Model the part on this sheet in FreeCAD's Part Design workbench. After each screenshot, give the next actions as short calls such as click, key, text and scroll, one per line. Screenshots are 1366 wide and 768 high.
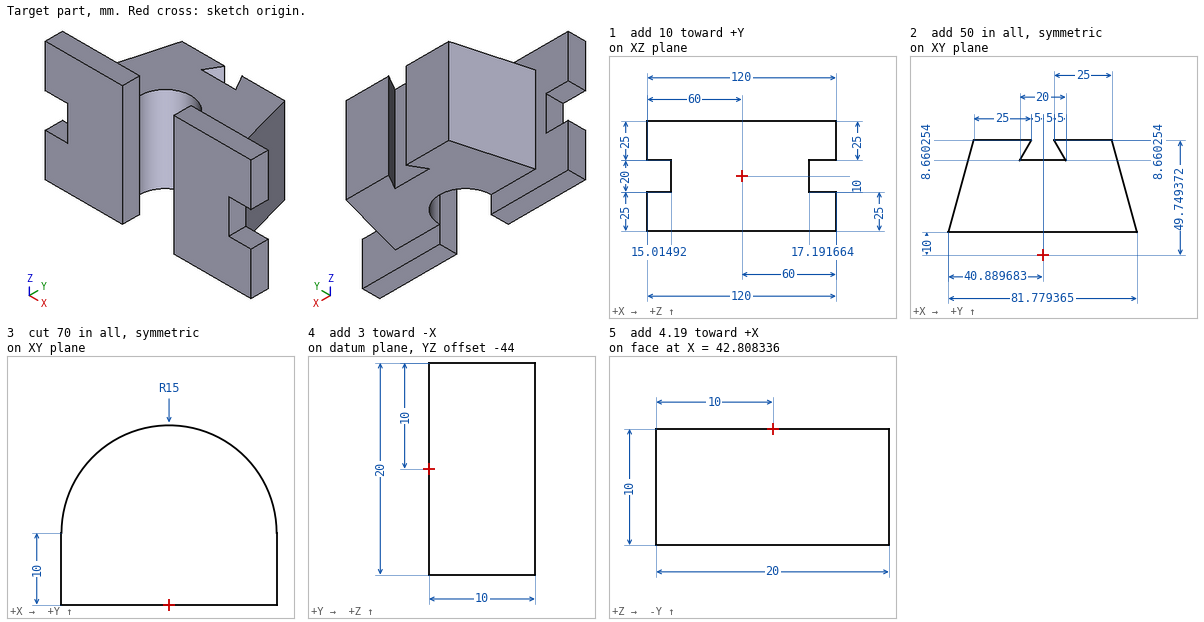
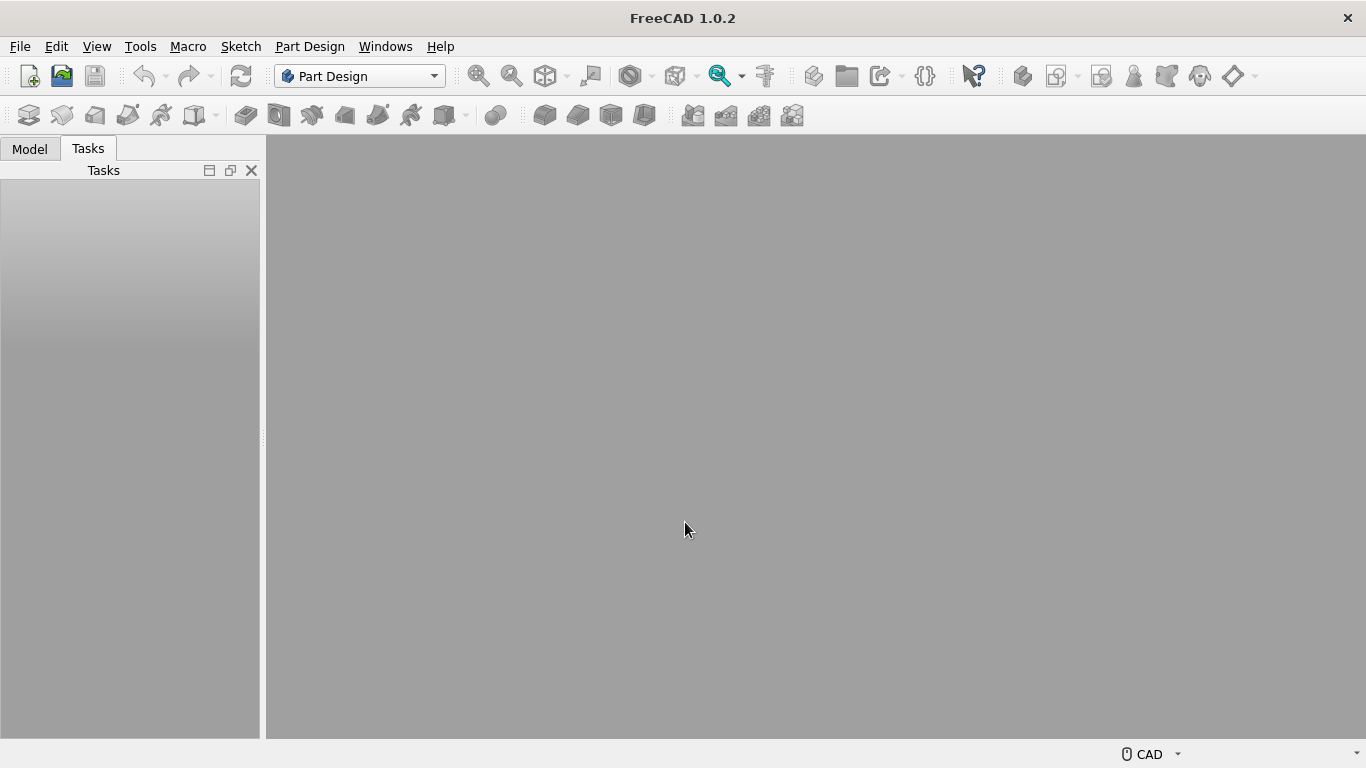
key(ctrl+n)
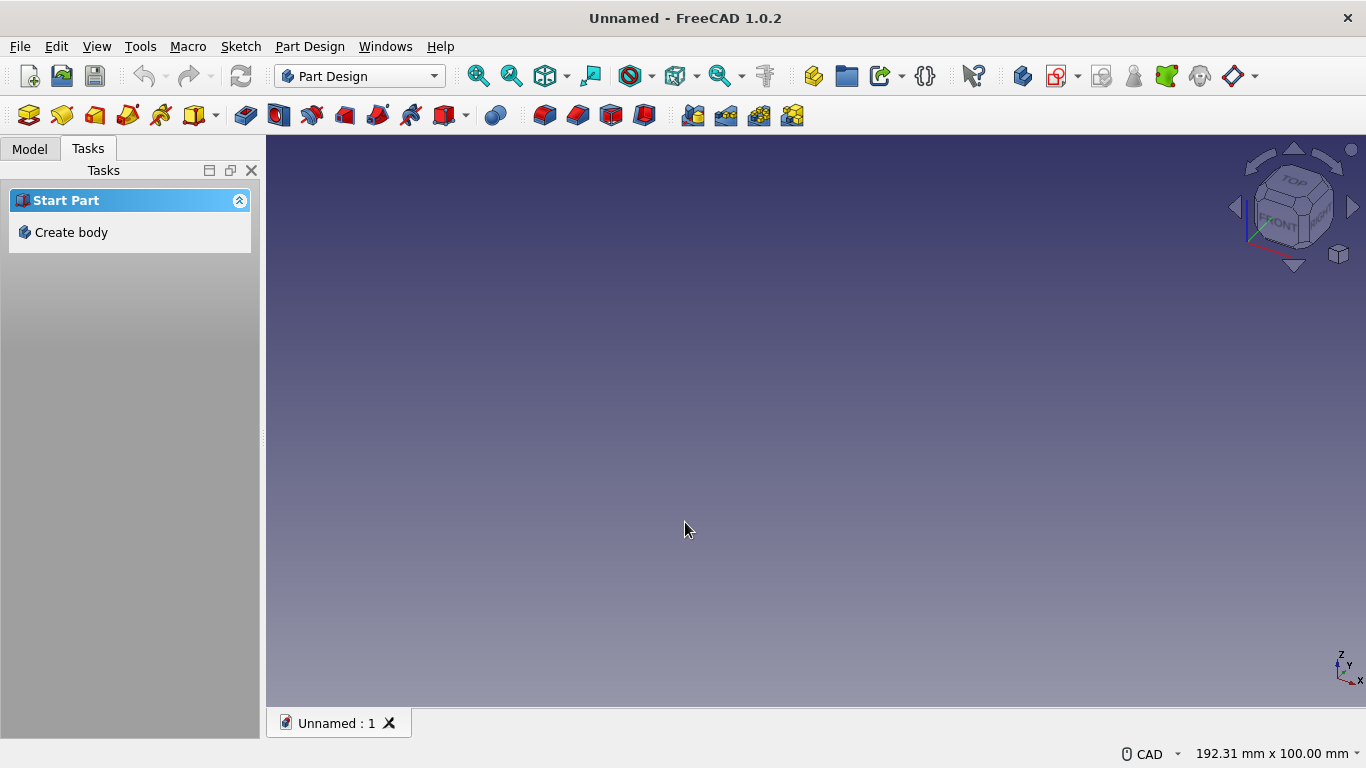
click(1056, 76)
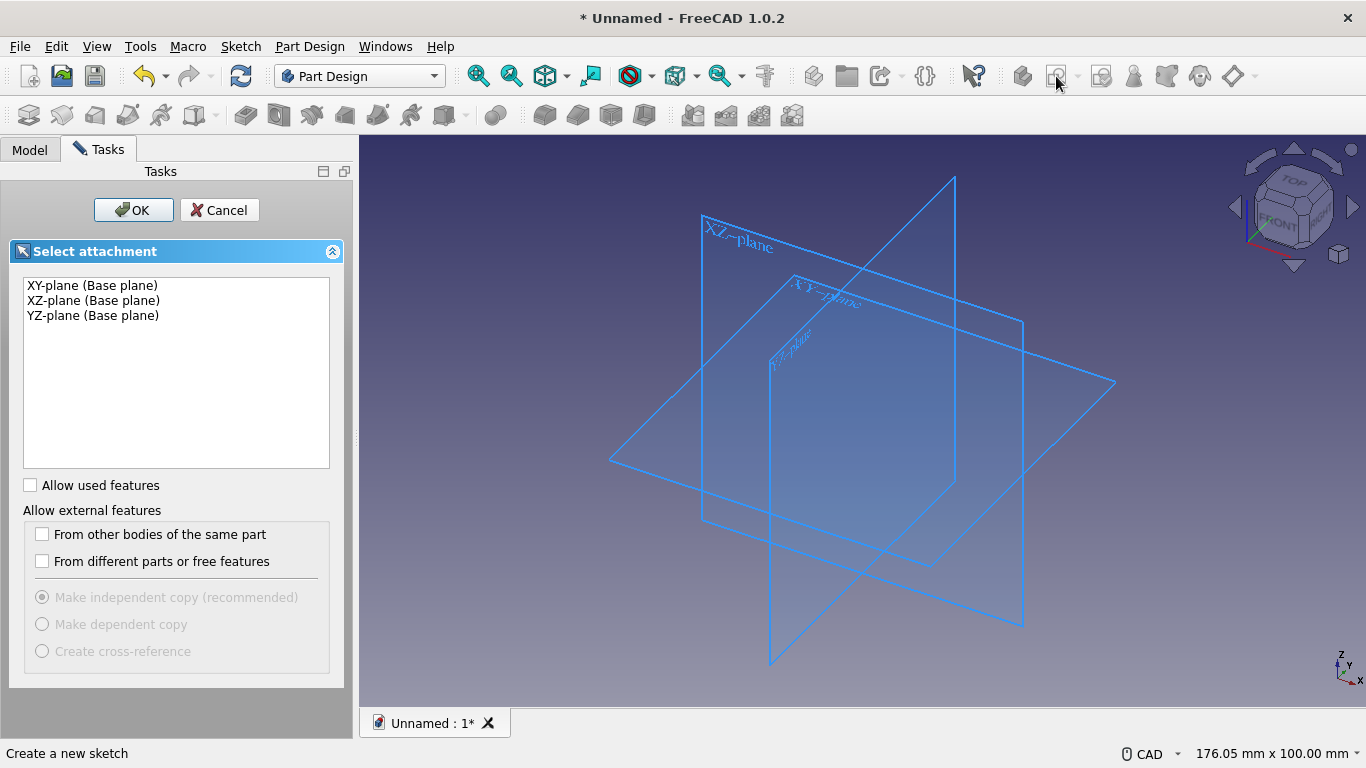
click(84, 300)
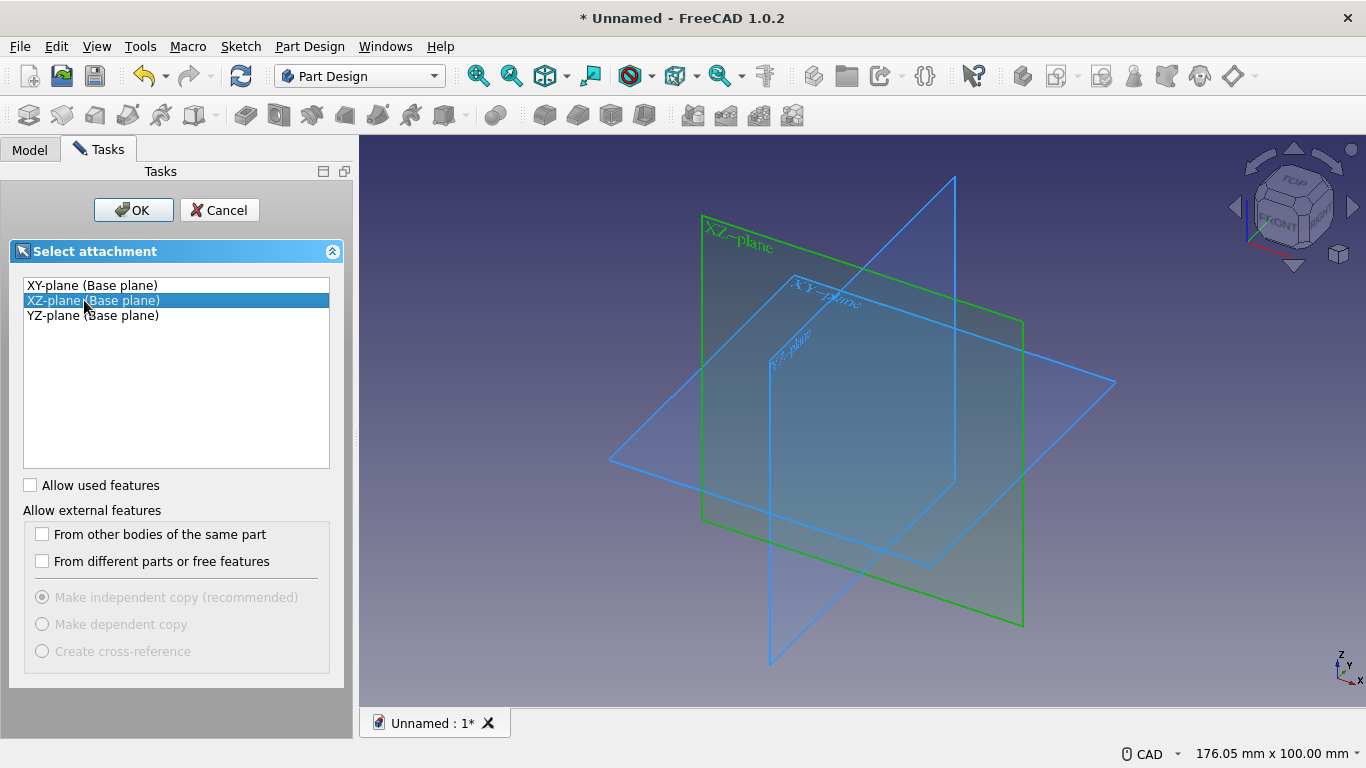
click(134, 210)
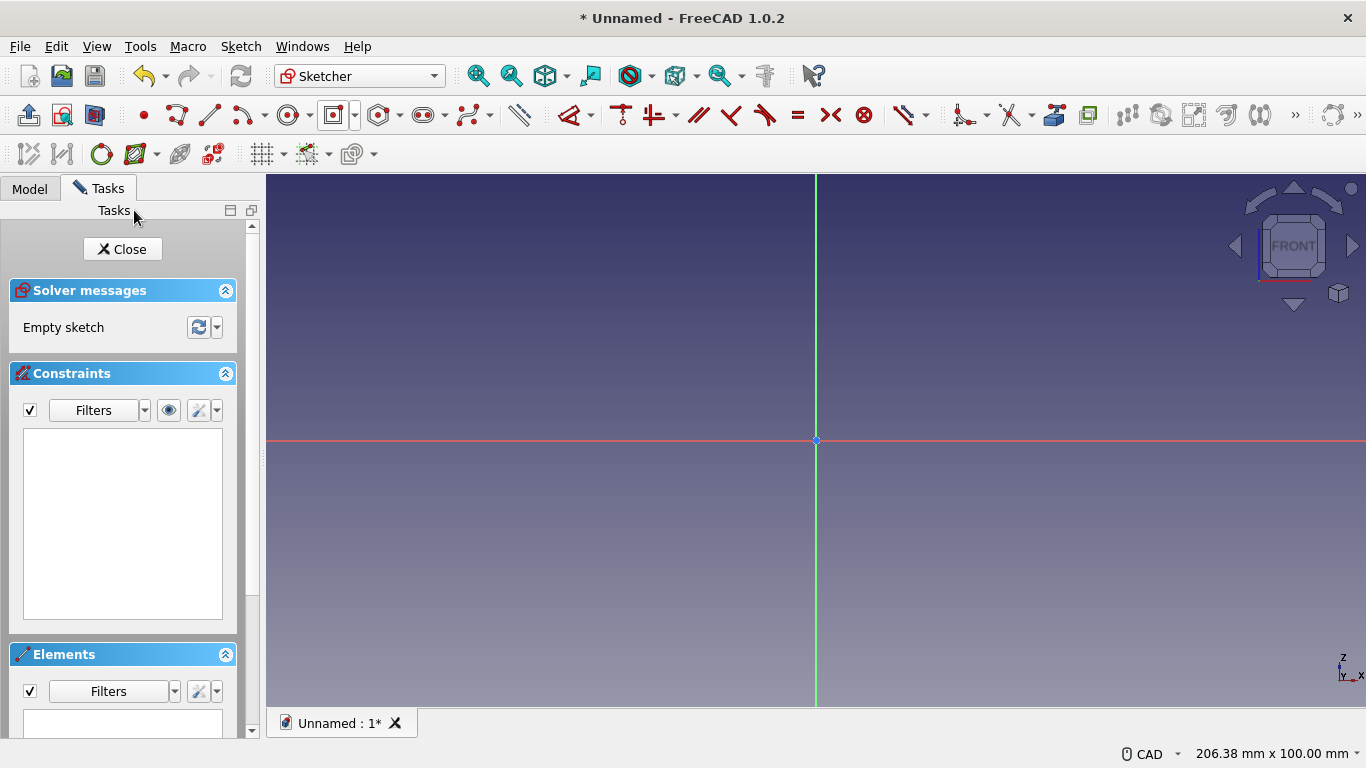
click(177, 116)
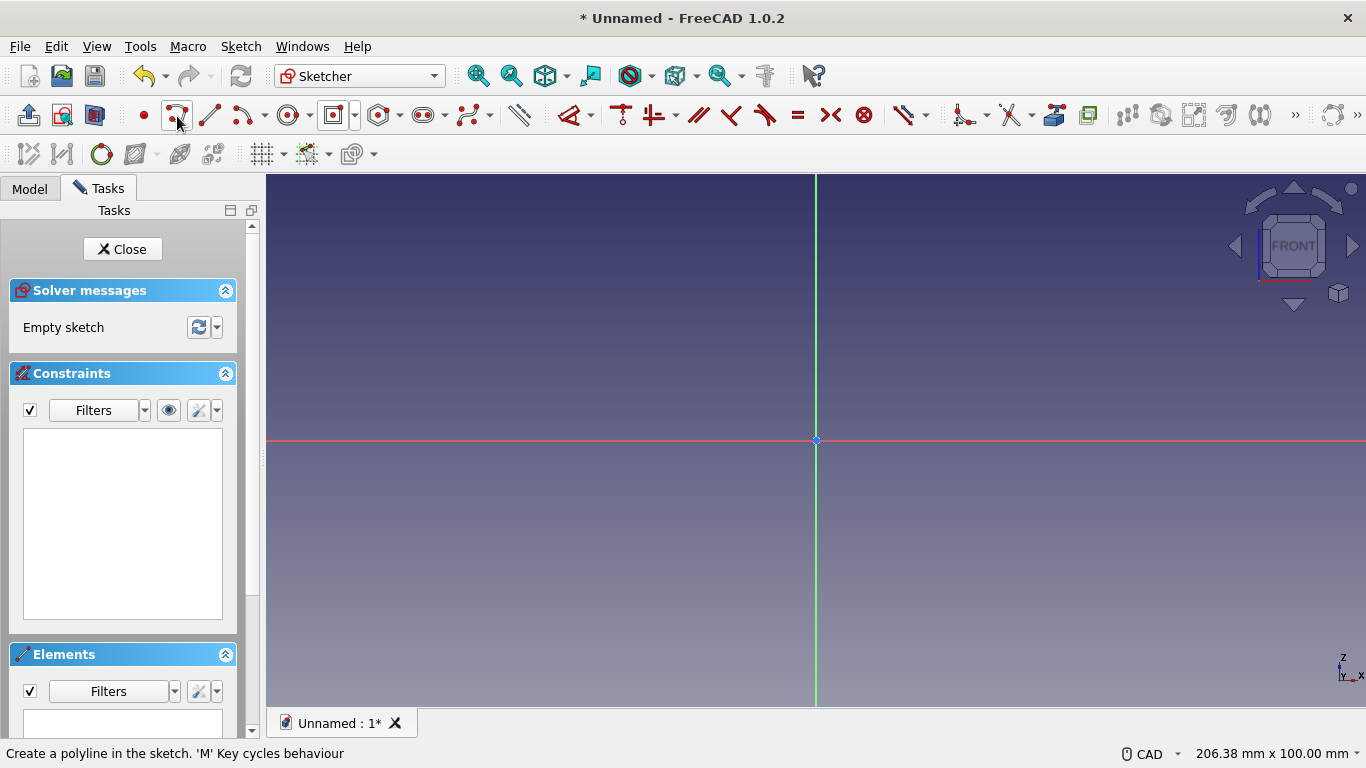
click(1044, 494)
click(1136, 494)
click(1136, 627)
click(496, 627)
click(496, 494)
click(576, 494)
click(576, 387)
click(496, 387)
click(496, 254)
click(1136, 254)
click(1136, 387)
click(1044, 387)
click(1044, 495)
key(Escape)
key(Escape)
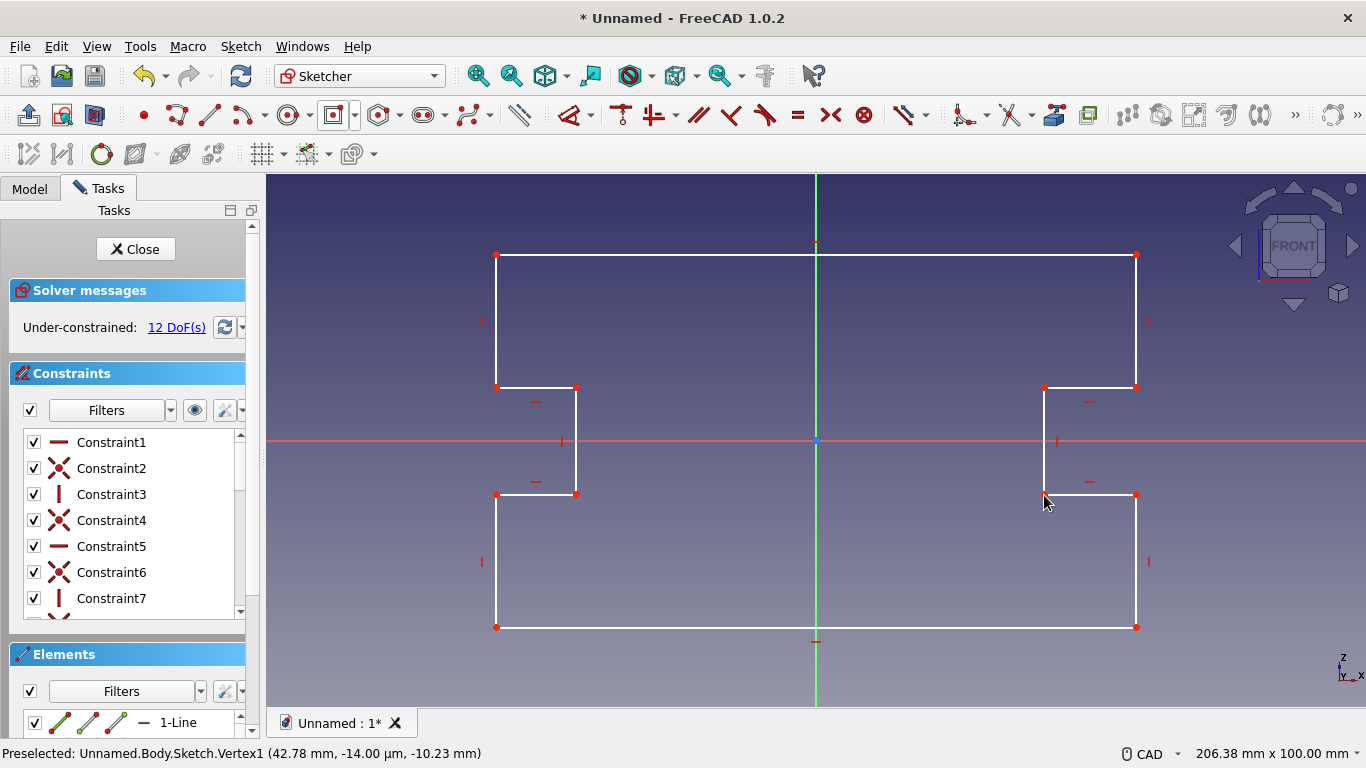
click(568, 116)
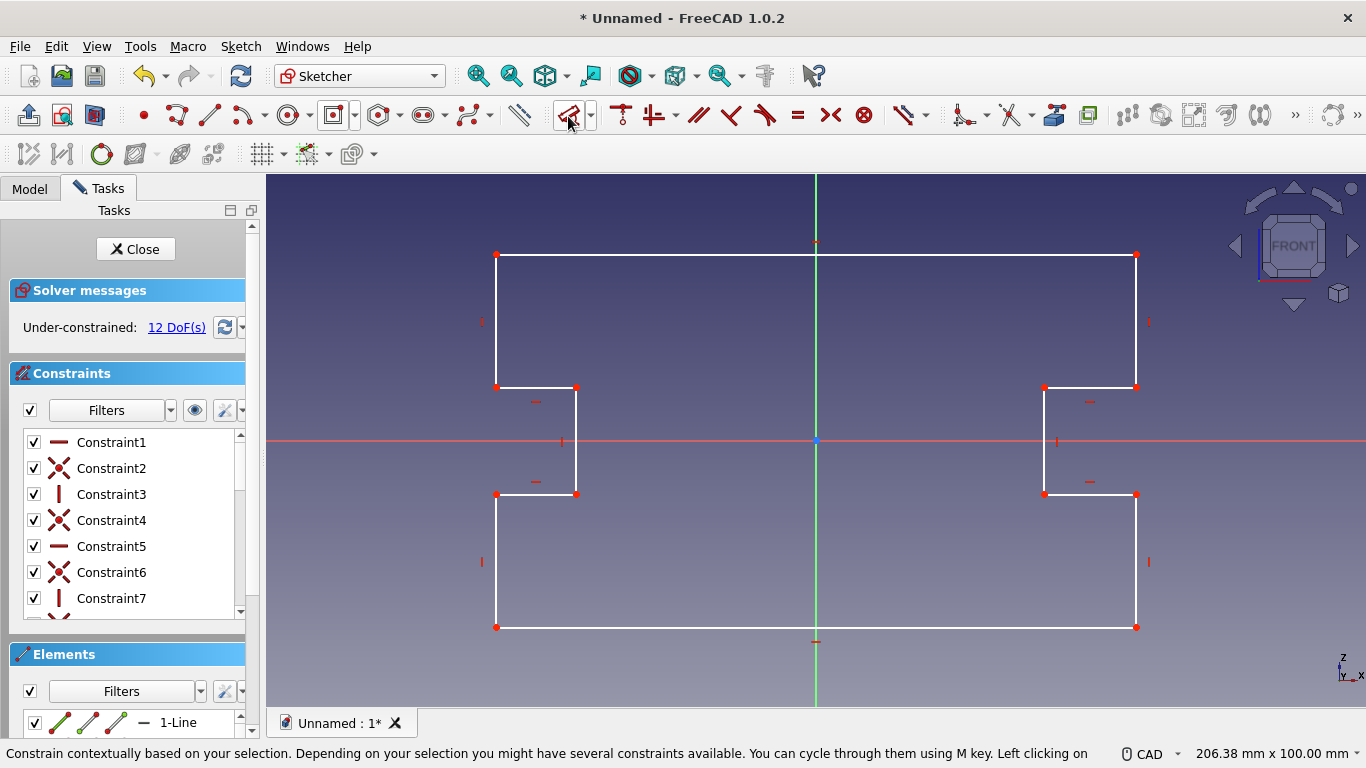
click(1136, 535)
click(1170, 562)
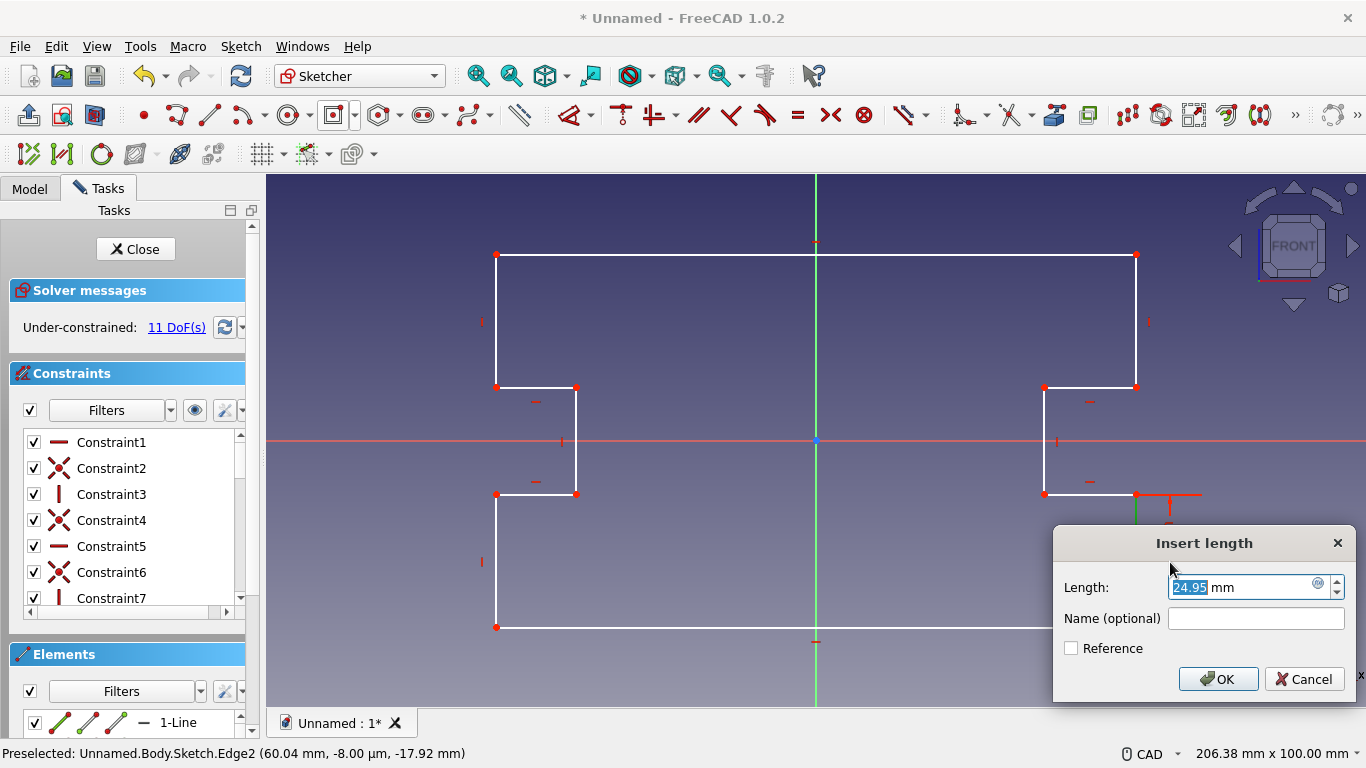
text(25)
key(Return)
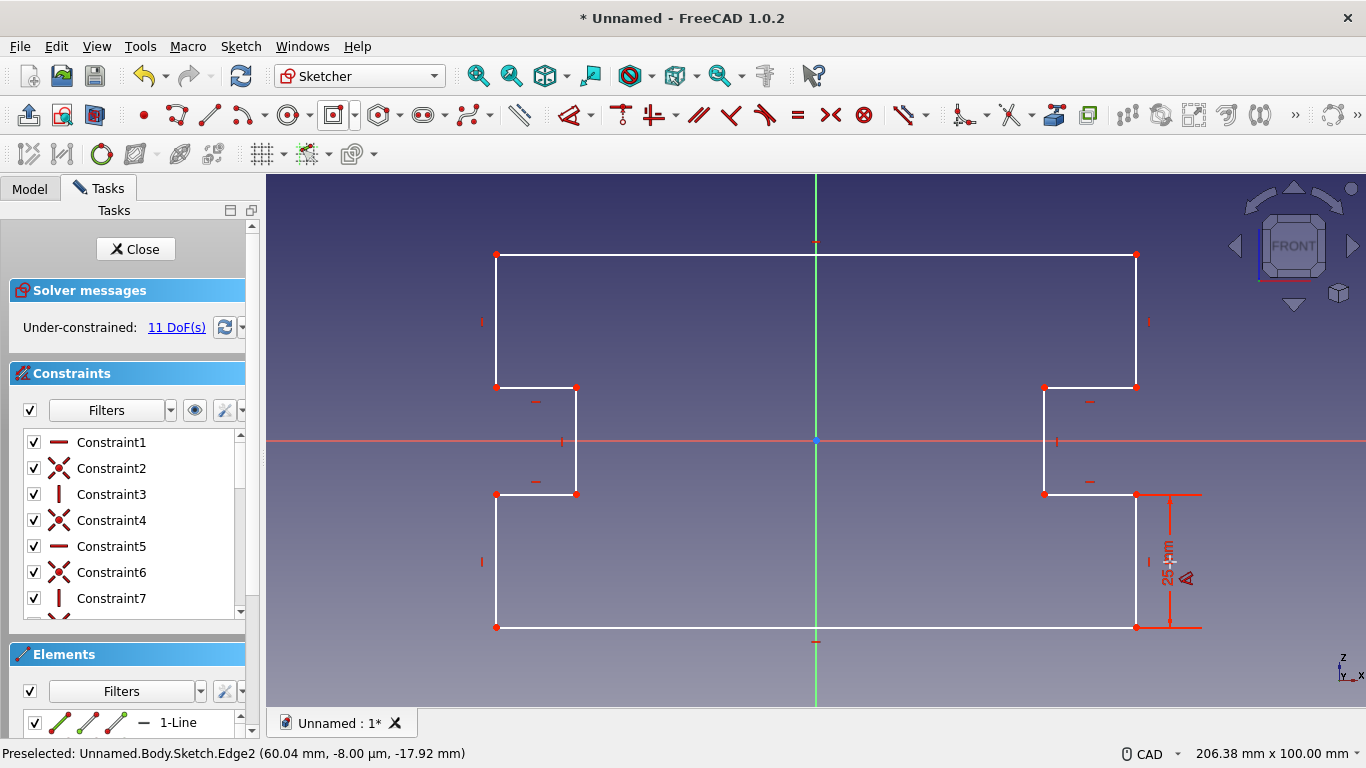
click(496, 588)
click(462, 562)